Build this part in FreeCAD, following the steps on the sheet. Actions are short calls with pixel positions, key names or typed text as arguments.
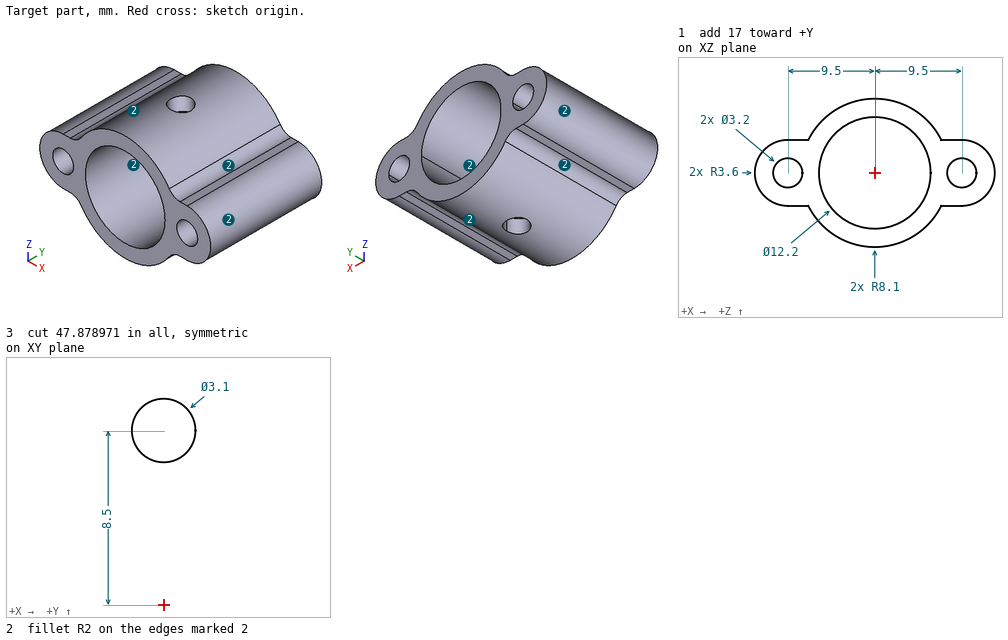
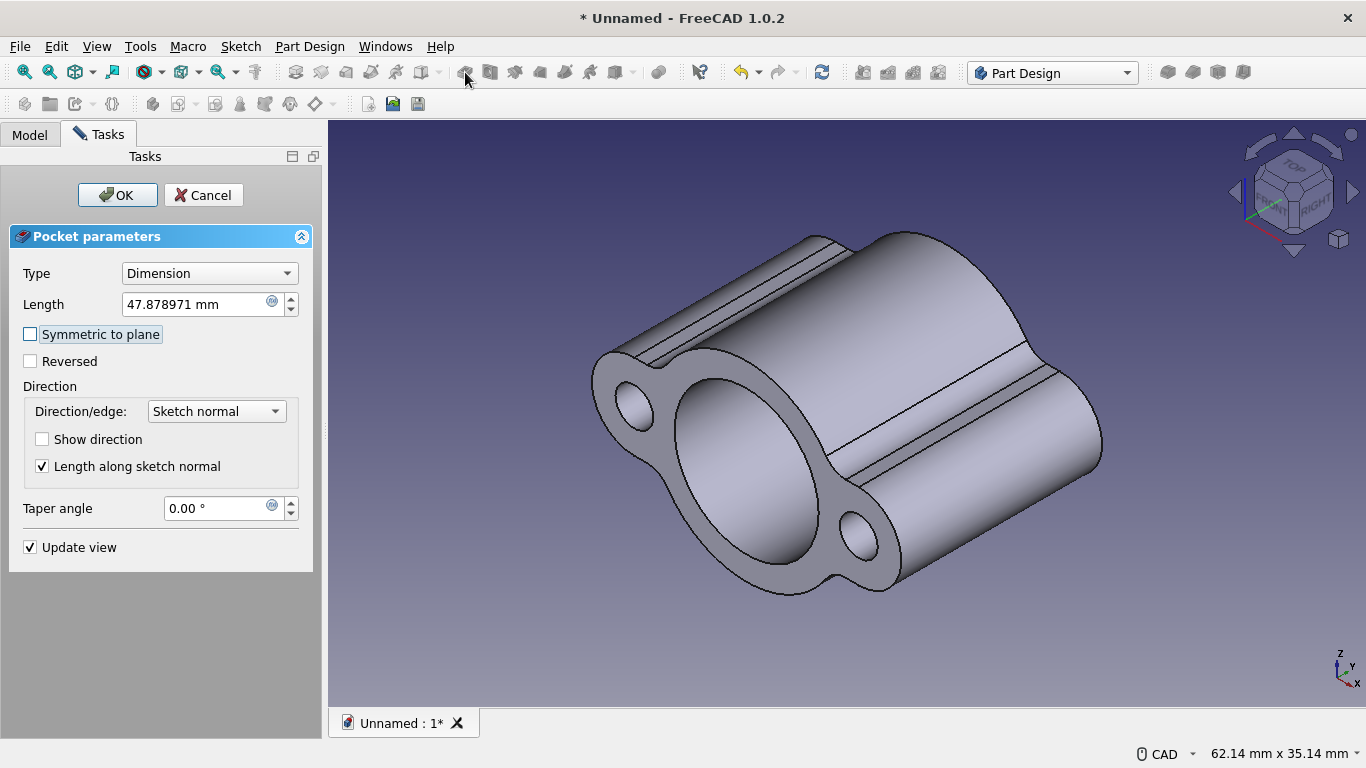
click(31, 334)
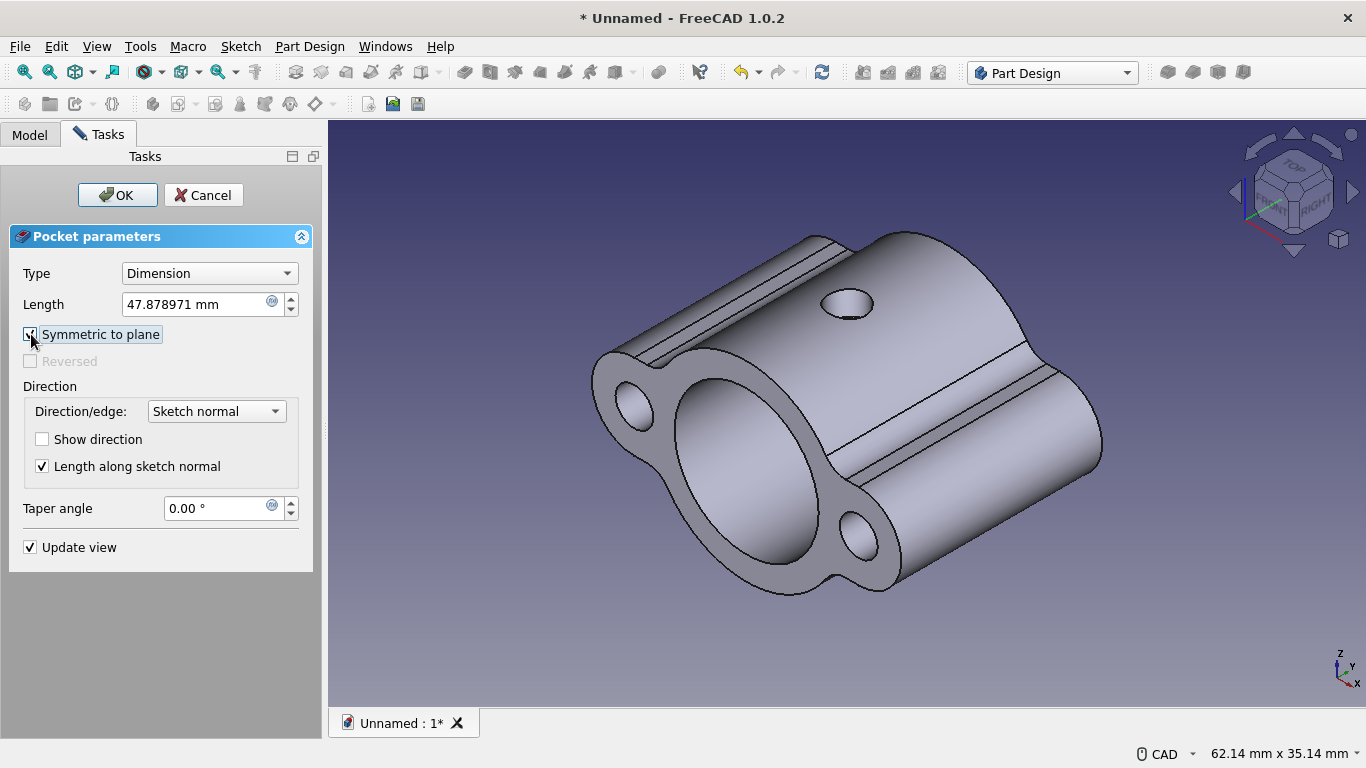
click(118, 195)